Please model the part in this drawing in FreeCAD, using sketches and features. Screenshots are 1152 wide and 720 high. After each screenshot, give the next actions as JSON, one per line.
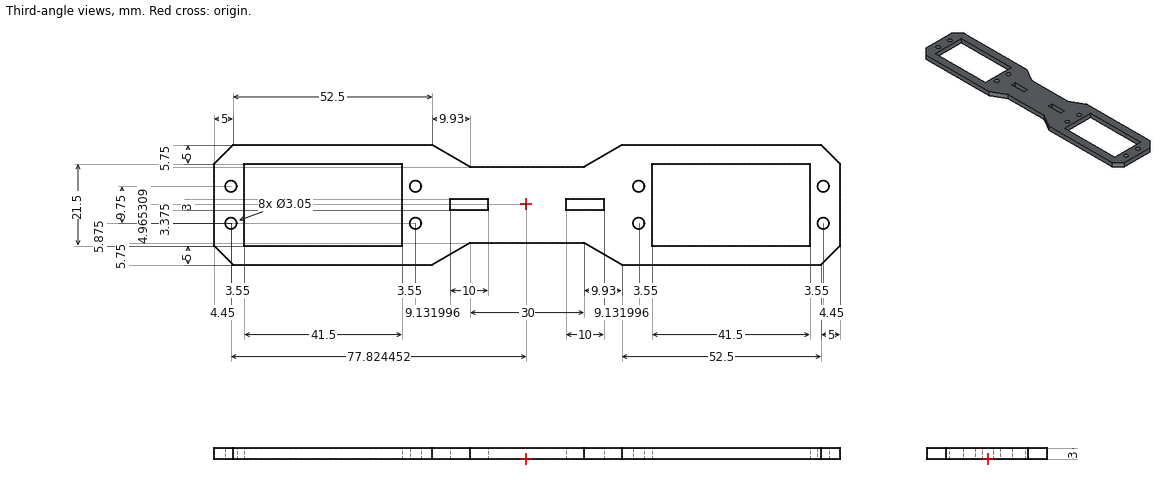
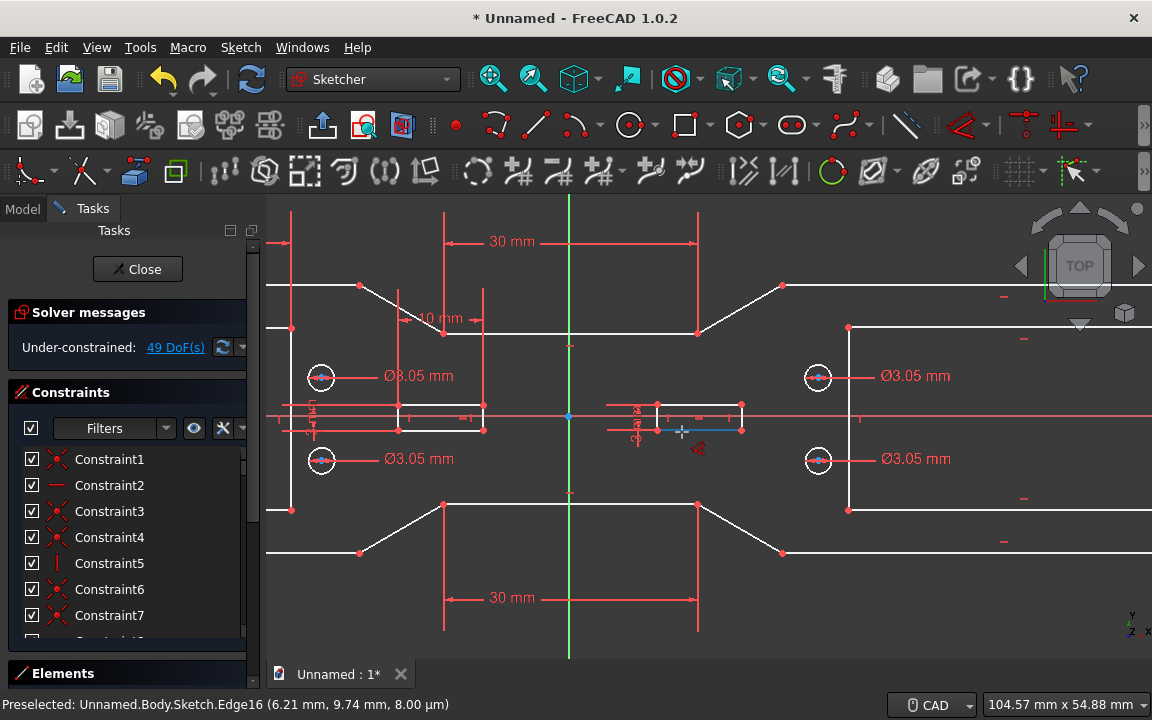
{"action": "left_click", "coordinate": [682, 430]}
{"action": "left_click", "coordinate": [699, 464]}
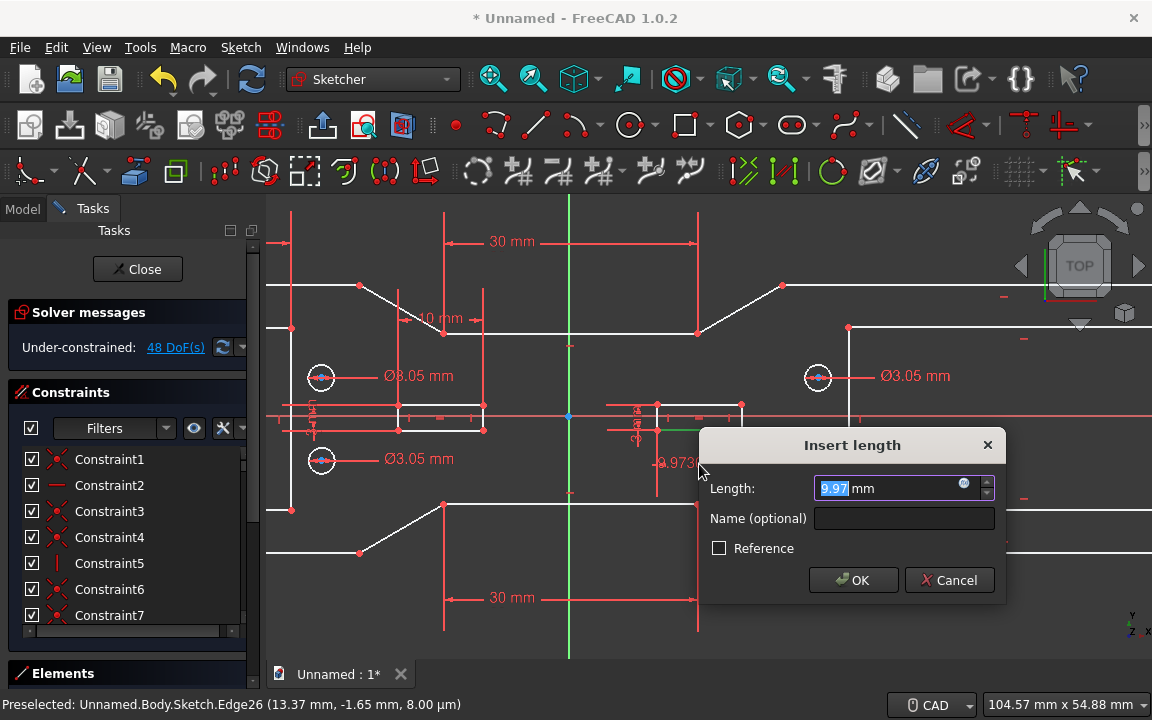
{"action": "type", "text": "10"}
{"action": "key", "text": "Return"}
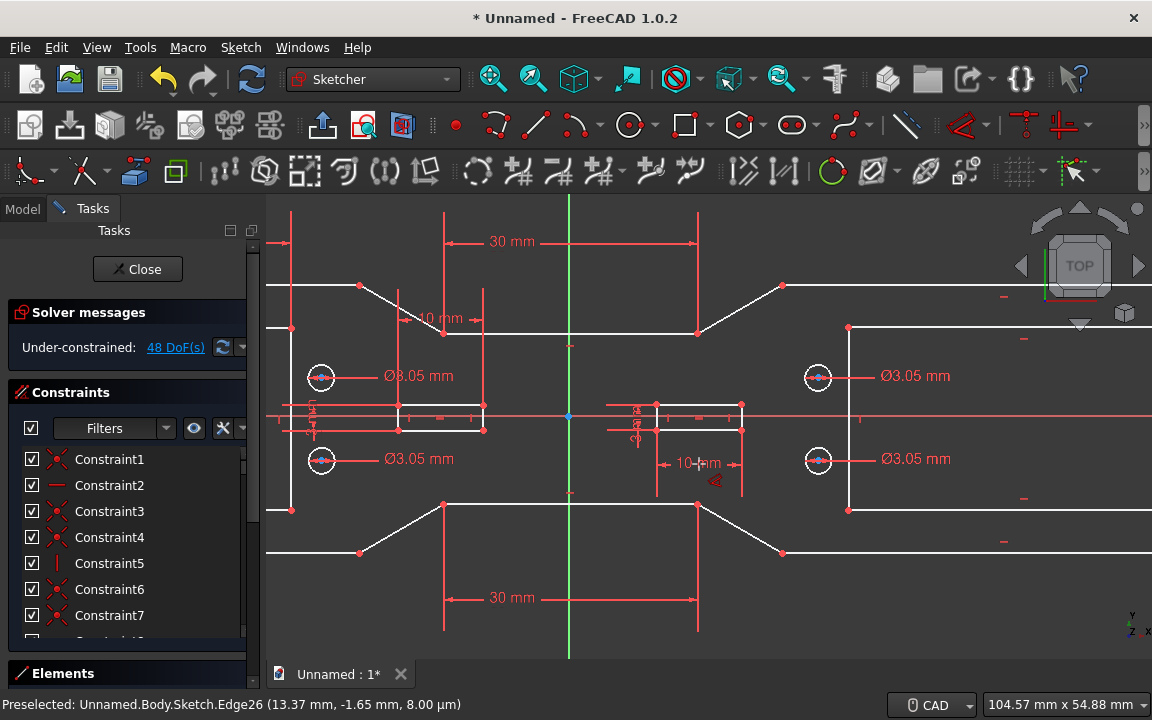
{"action": "scroll", "coordinate": [681, 432], "scroll_direction": "down", "scroll_amount": 5}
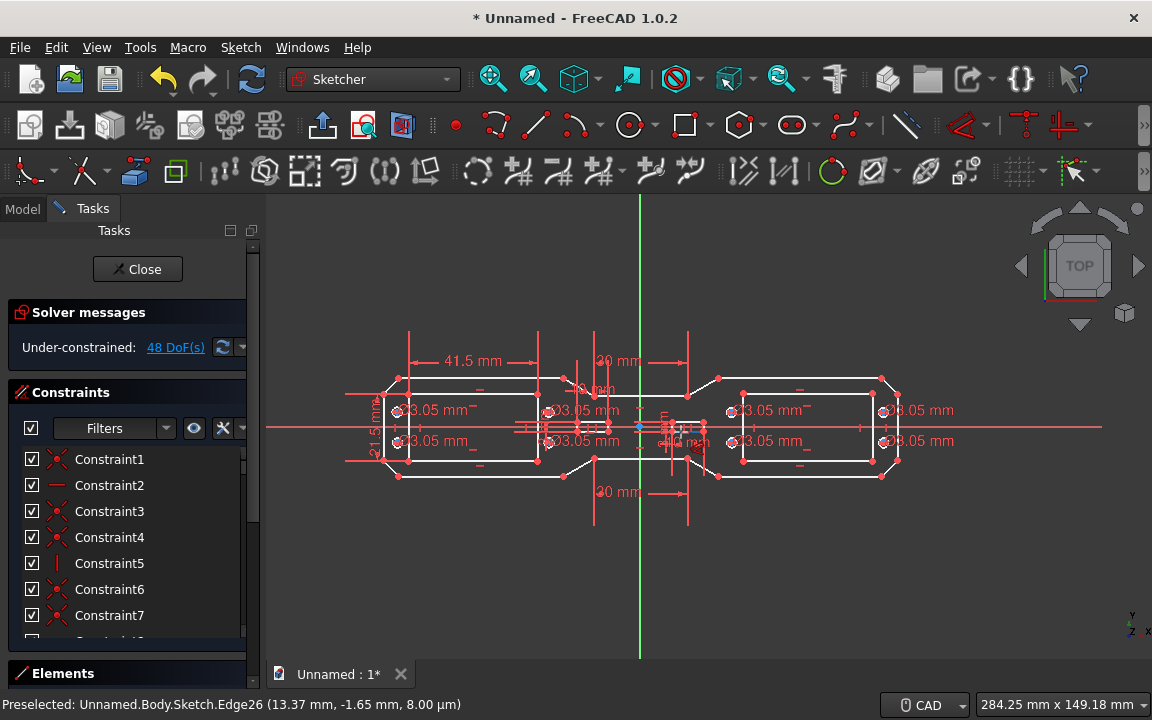
{"action": "scroll", "coordinate": [394, 383], "scroll_direction": "up", "scroll_amount": 5}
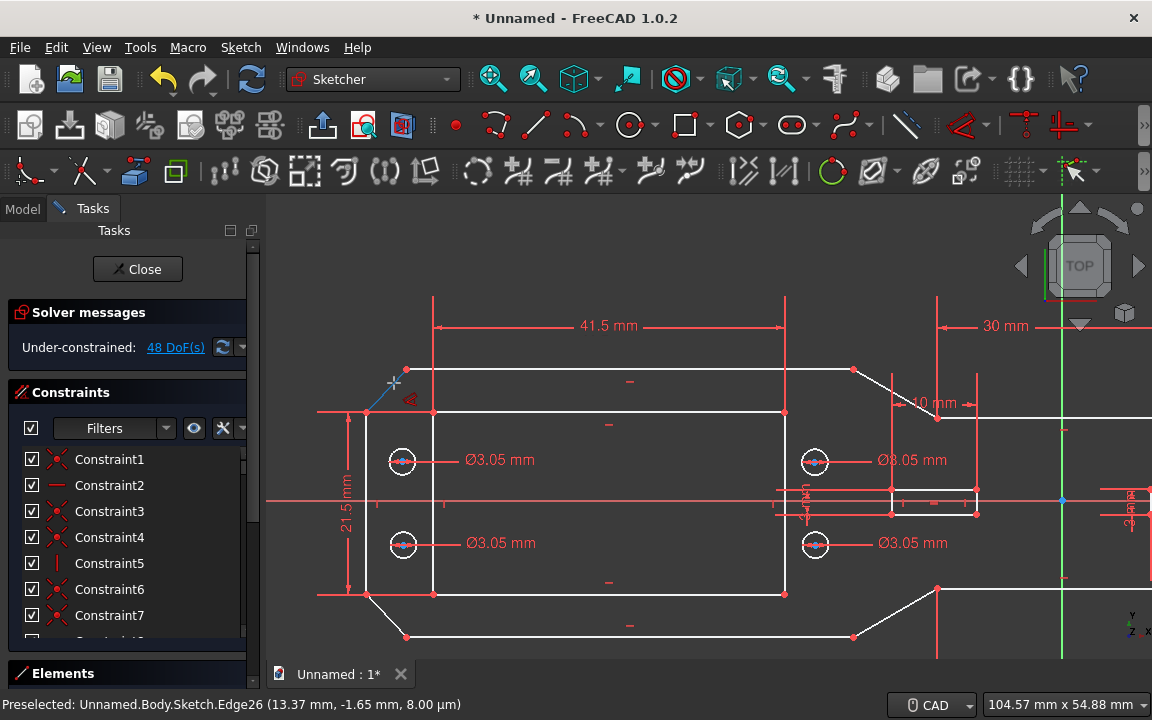
{"action": "left_click", "coordinate": [395, 382]}
{"action": "left_click", "coordinate": [387, 335]}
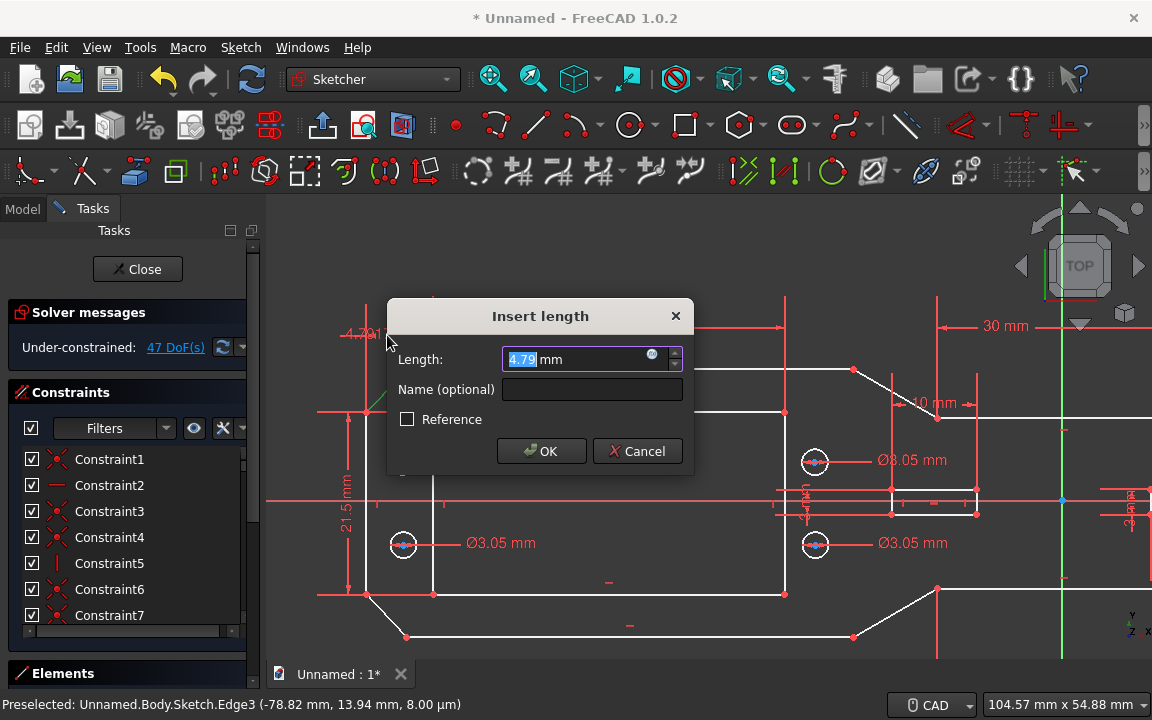
{"action": "type", "text": "5"}
{"action": "key", "text": "Return"}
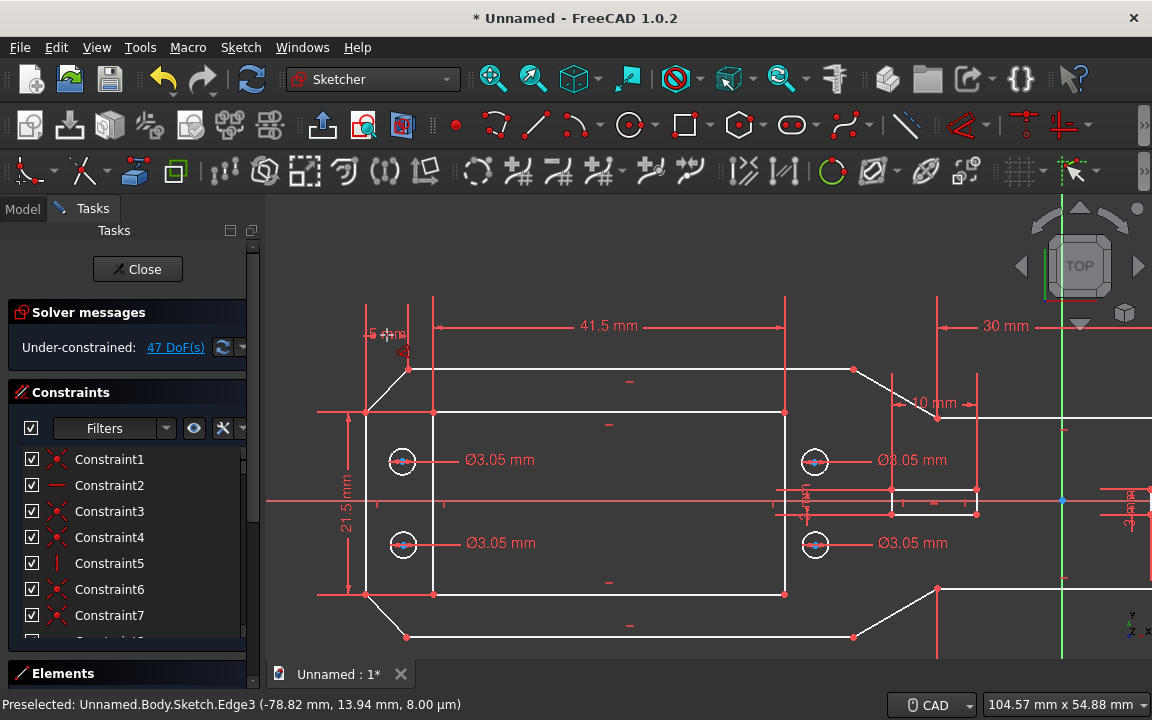
{"action": "left_click", "coordinate": [395, 382]}
{"action": "left_click", "coordinate": [332, 391]}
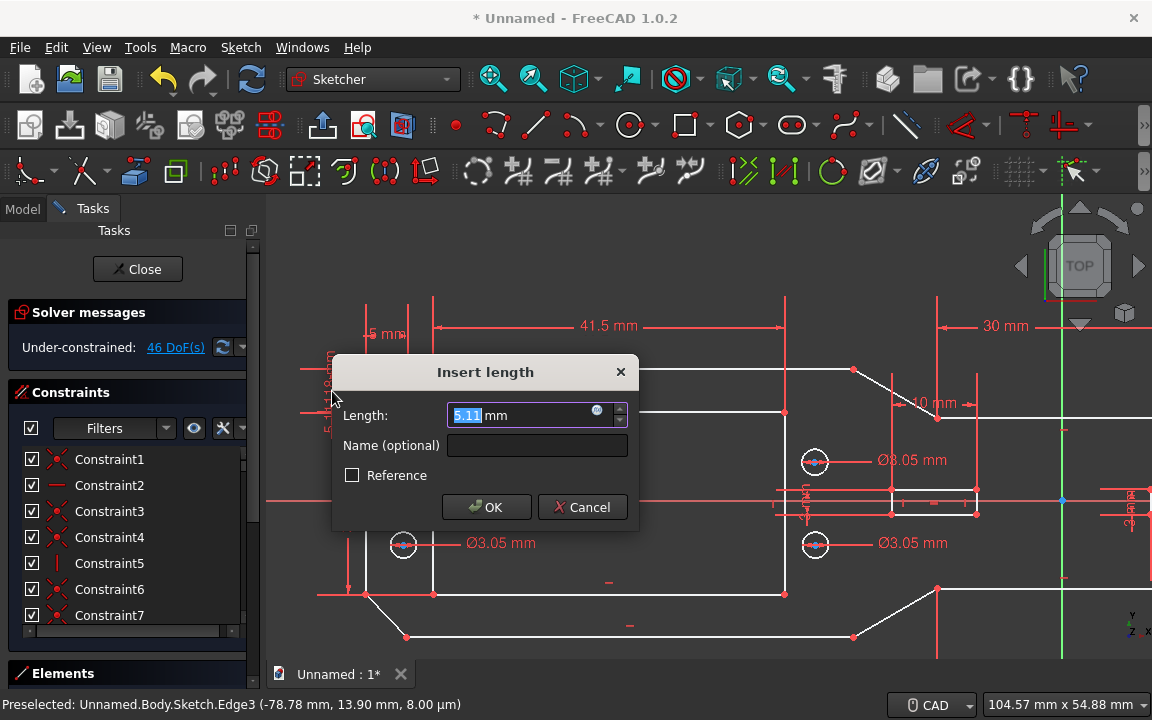
{"action": "type", "text": "5"}
{"action": "key", "text": "Return"}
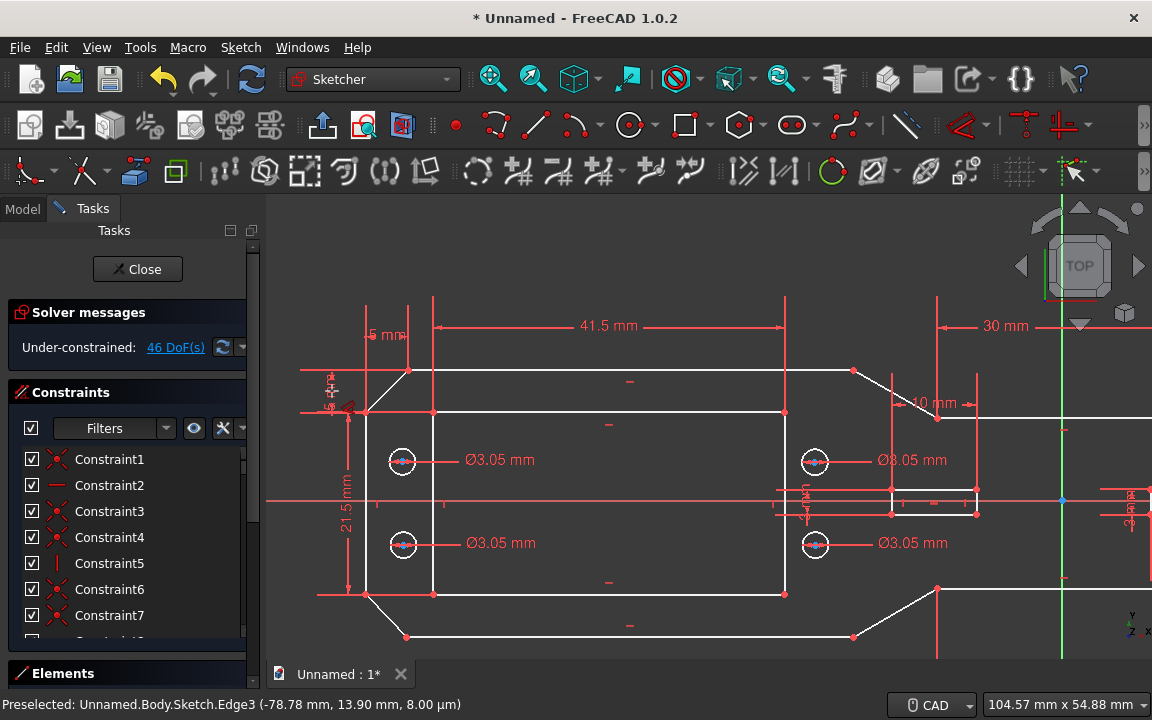
{"action": "left_click", "coordinate": [378, 607]}
{"action": "left_click", "coordinate": [386, 440]}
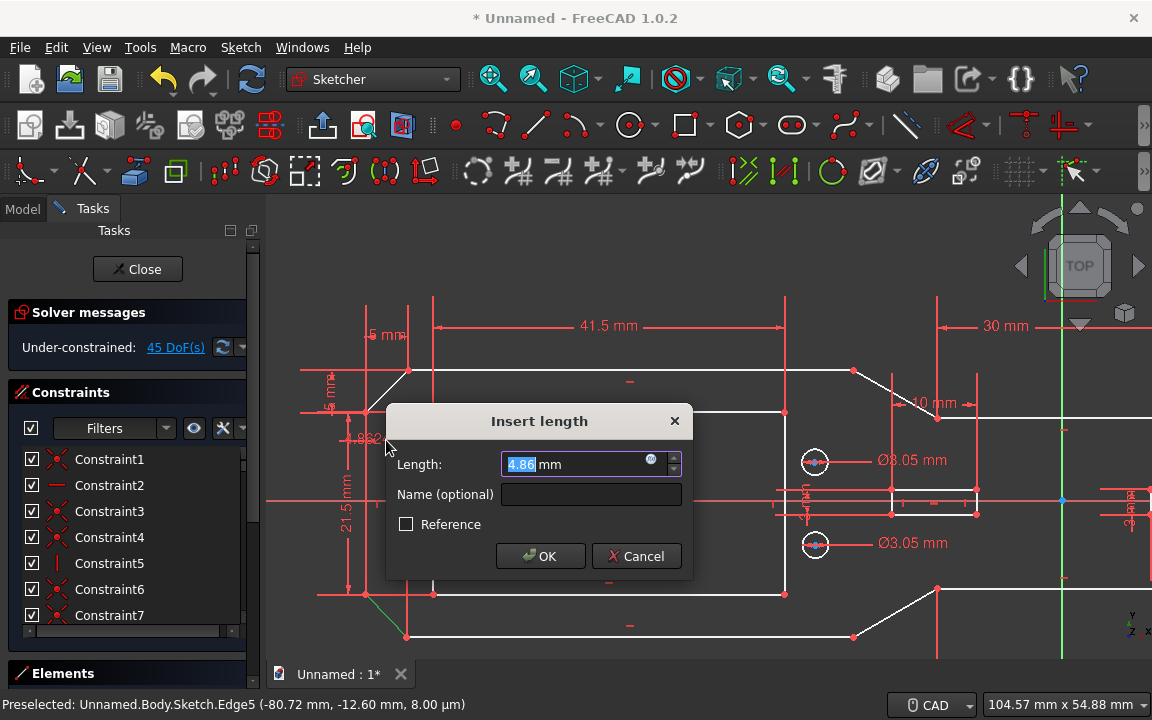
{"action": "type", "text": "5"}
{"action": "key", "text": "Return"}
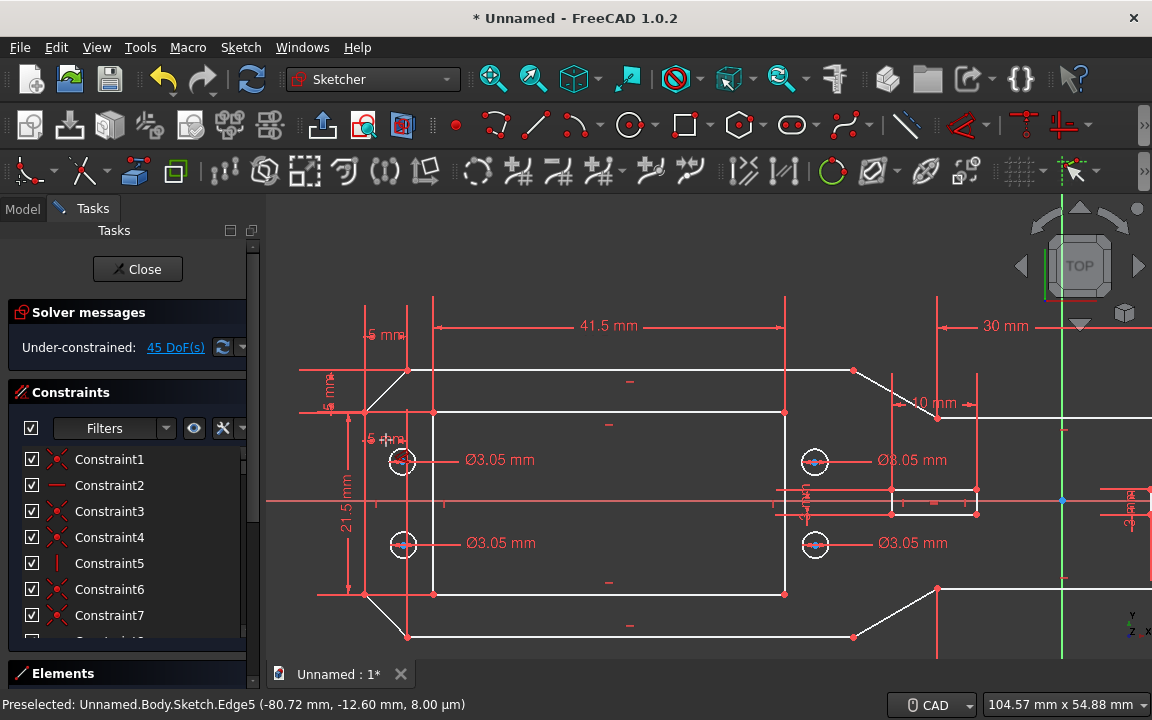
{"action": "left_click", "coordinate": [378, 607]}
{"action": "left_click", "coordinate": [331, 613]}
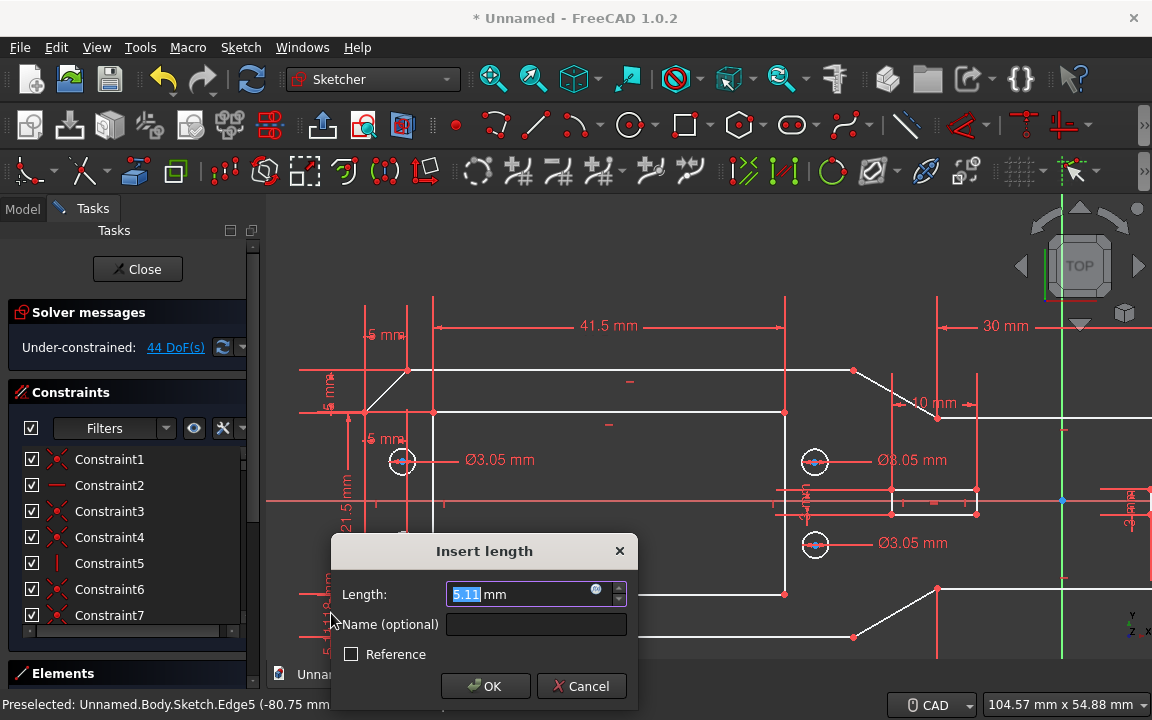
{"action": "type", "text": "5"}
{"action": "key", "text": "Return"}